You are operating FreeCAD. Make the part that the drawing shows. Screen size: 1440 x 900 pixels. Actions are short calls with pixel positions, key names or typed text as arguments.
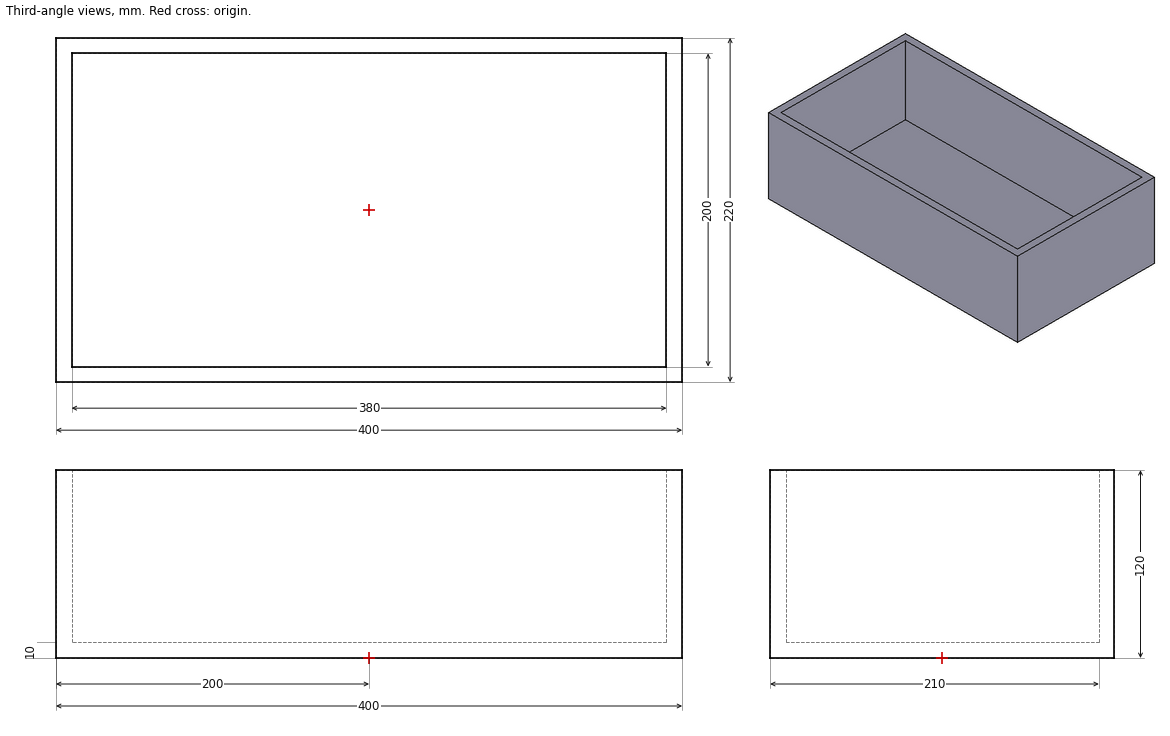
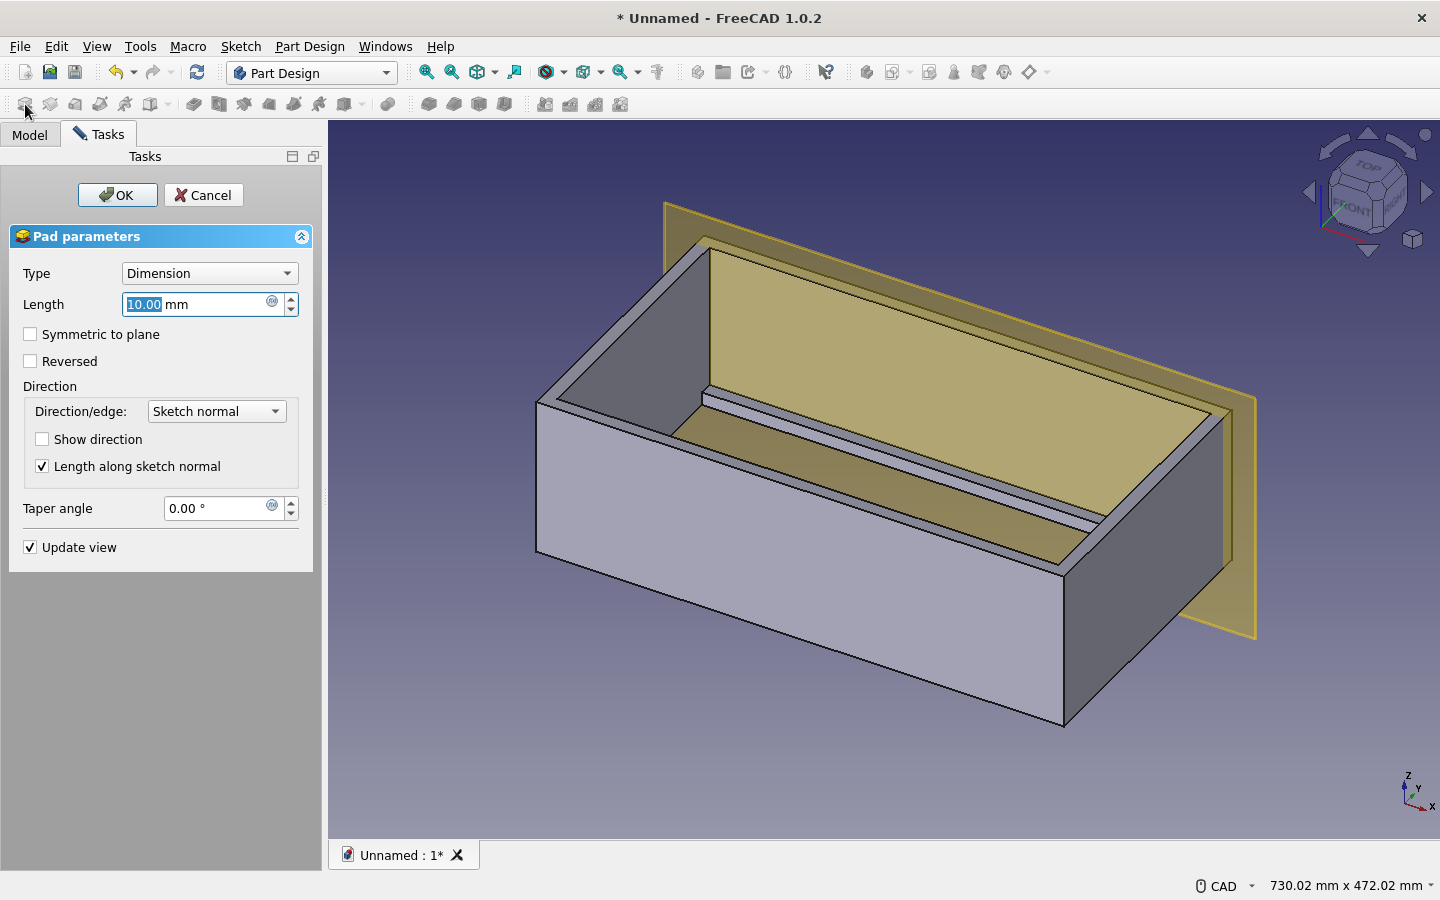
text(210)
key(Tab)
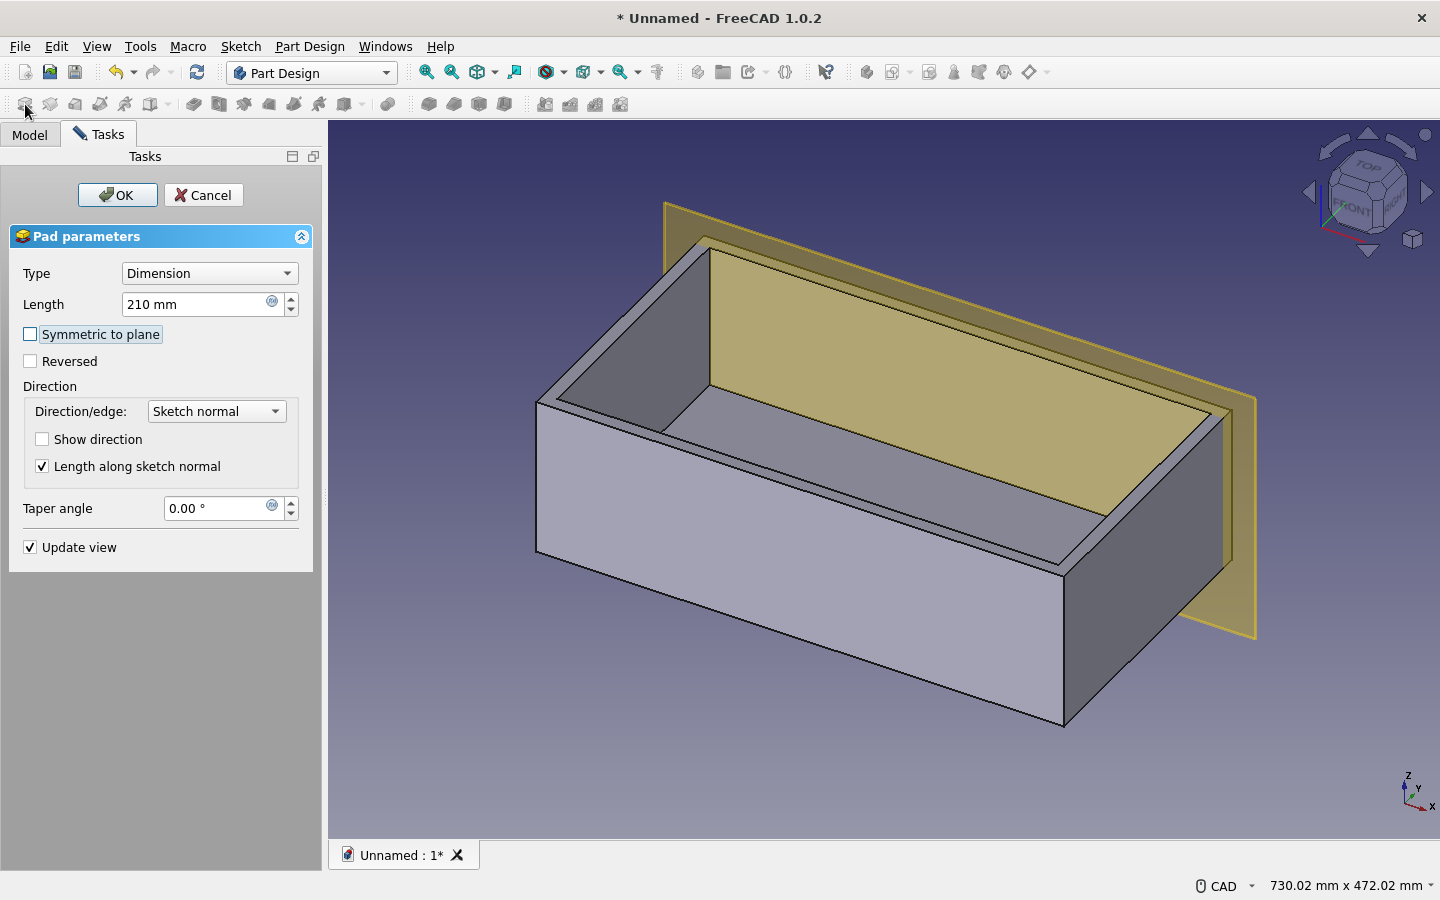
click(118, 195)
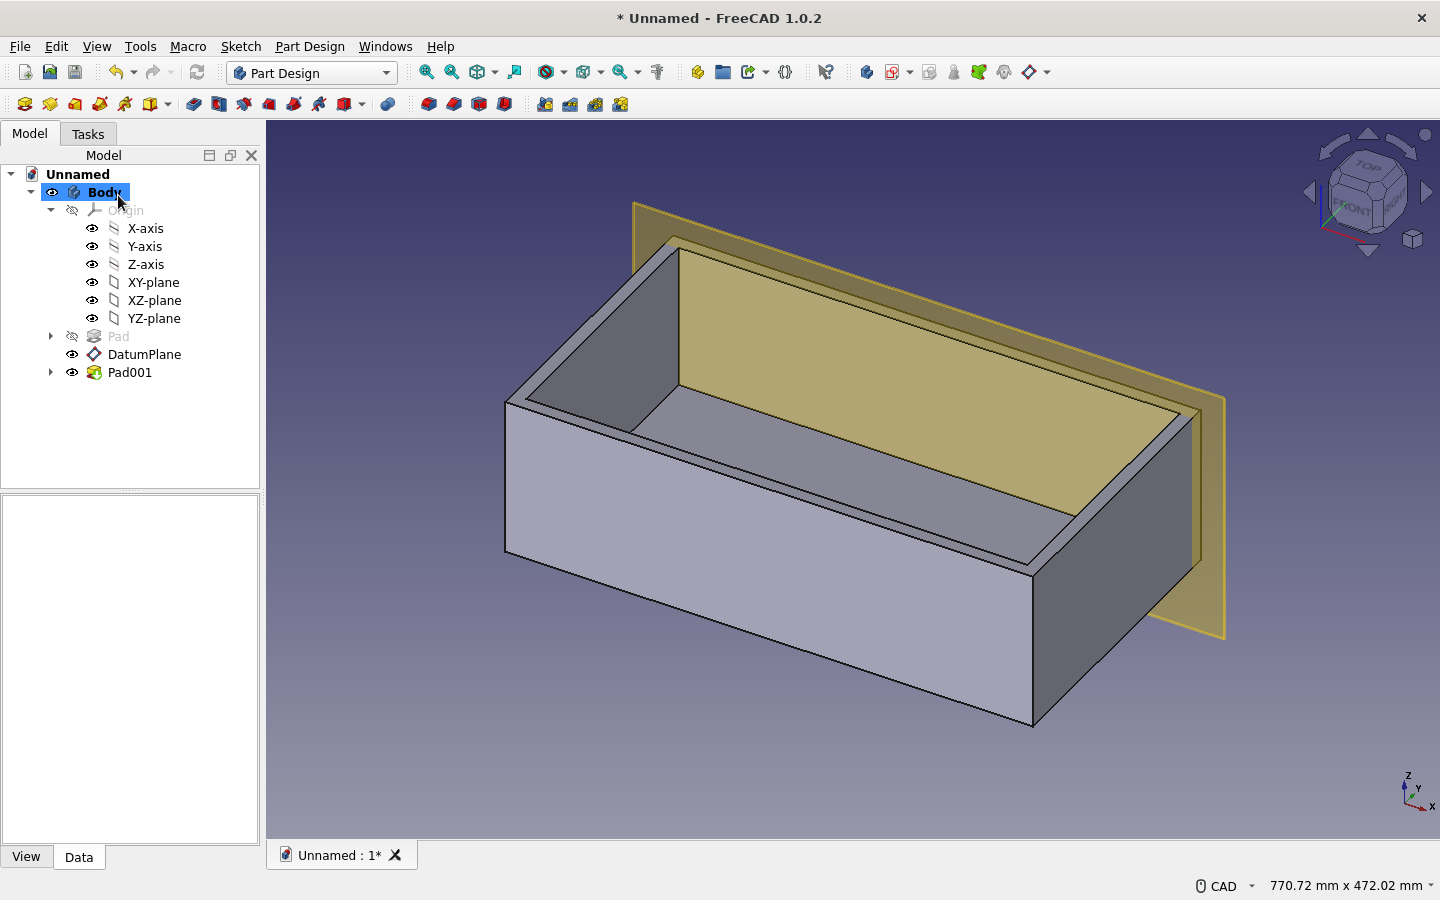
click(117, 354)
key(space)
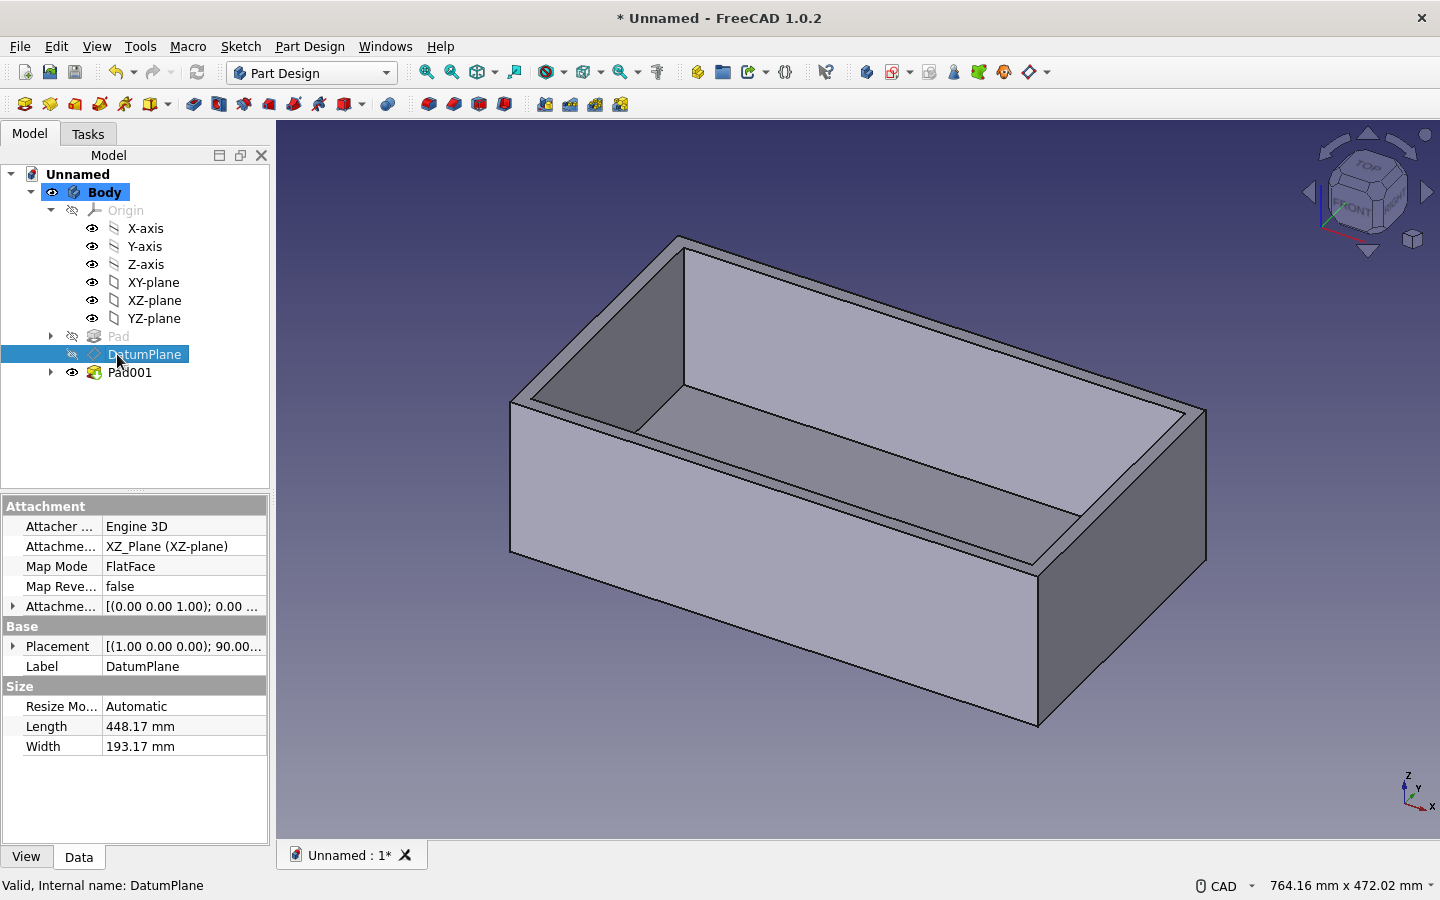
key(0)